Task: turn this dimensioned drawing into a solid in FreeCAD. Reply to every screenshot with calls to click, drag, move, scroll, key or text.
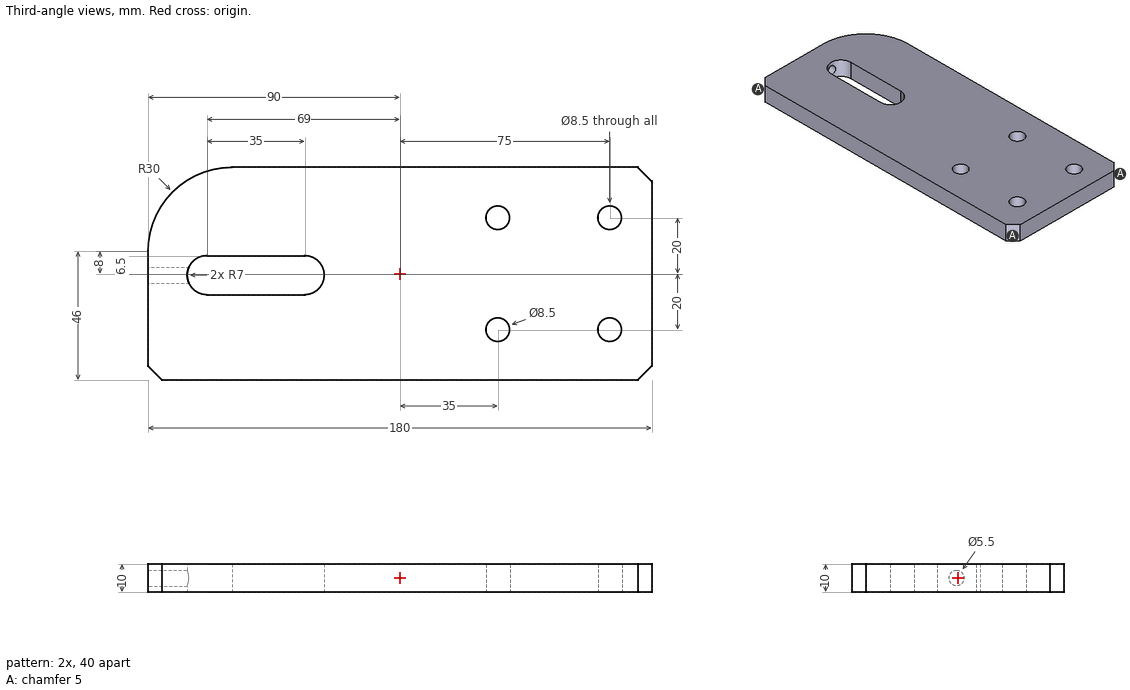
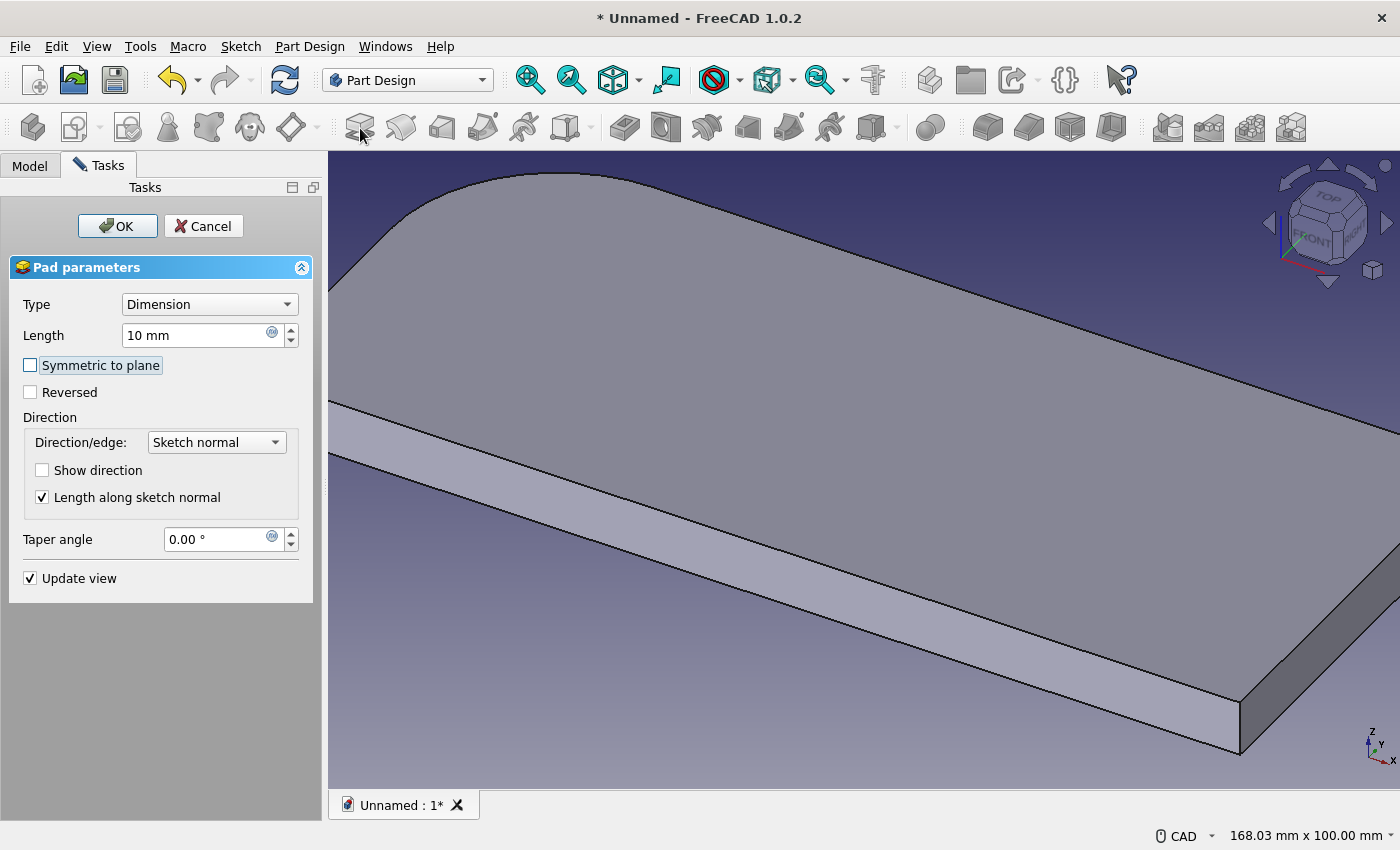
click(31, 365)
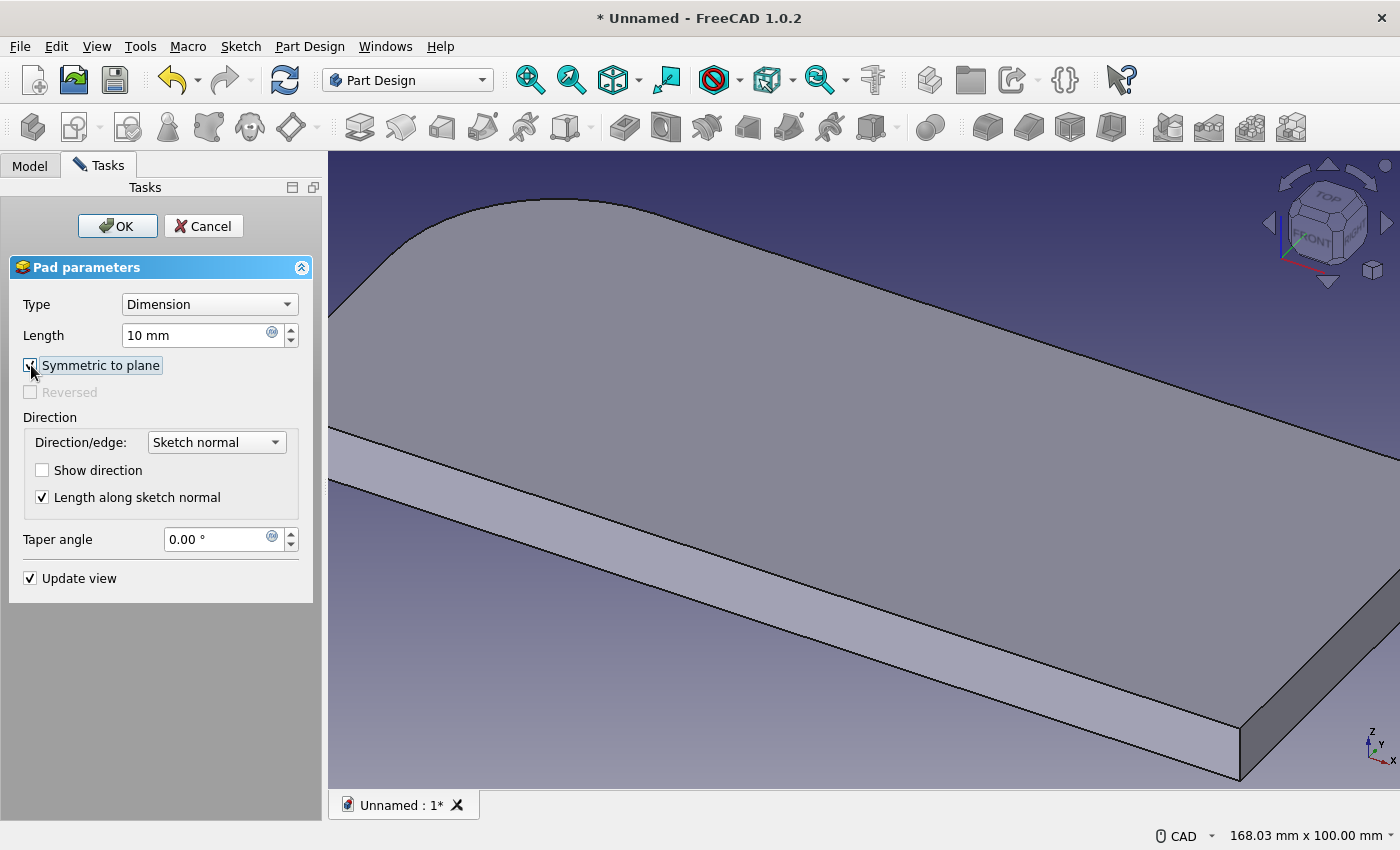
click(118, 226)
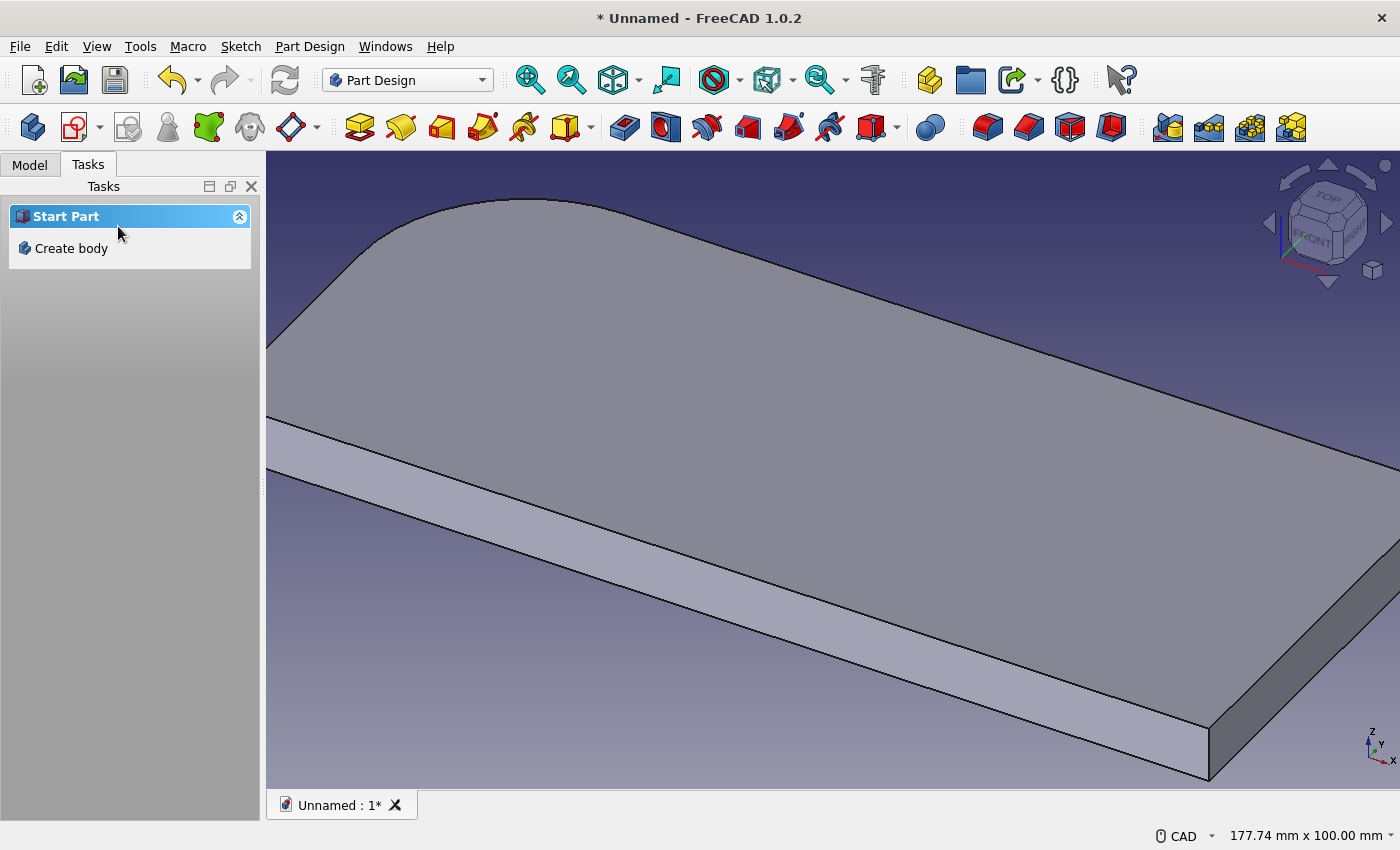
click(531, 80)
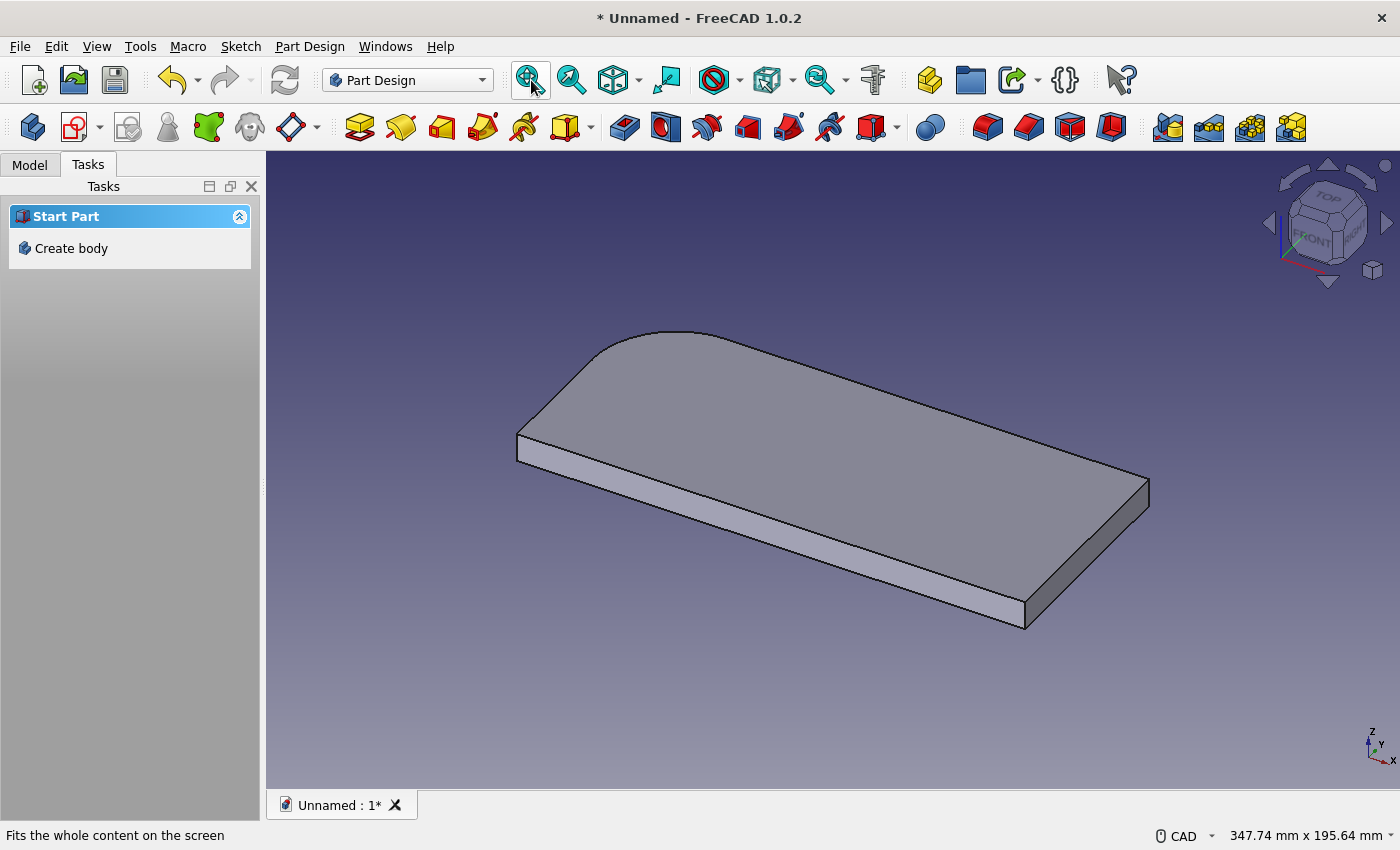
click(978, 504)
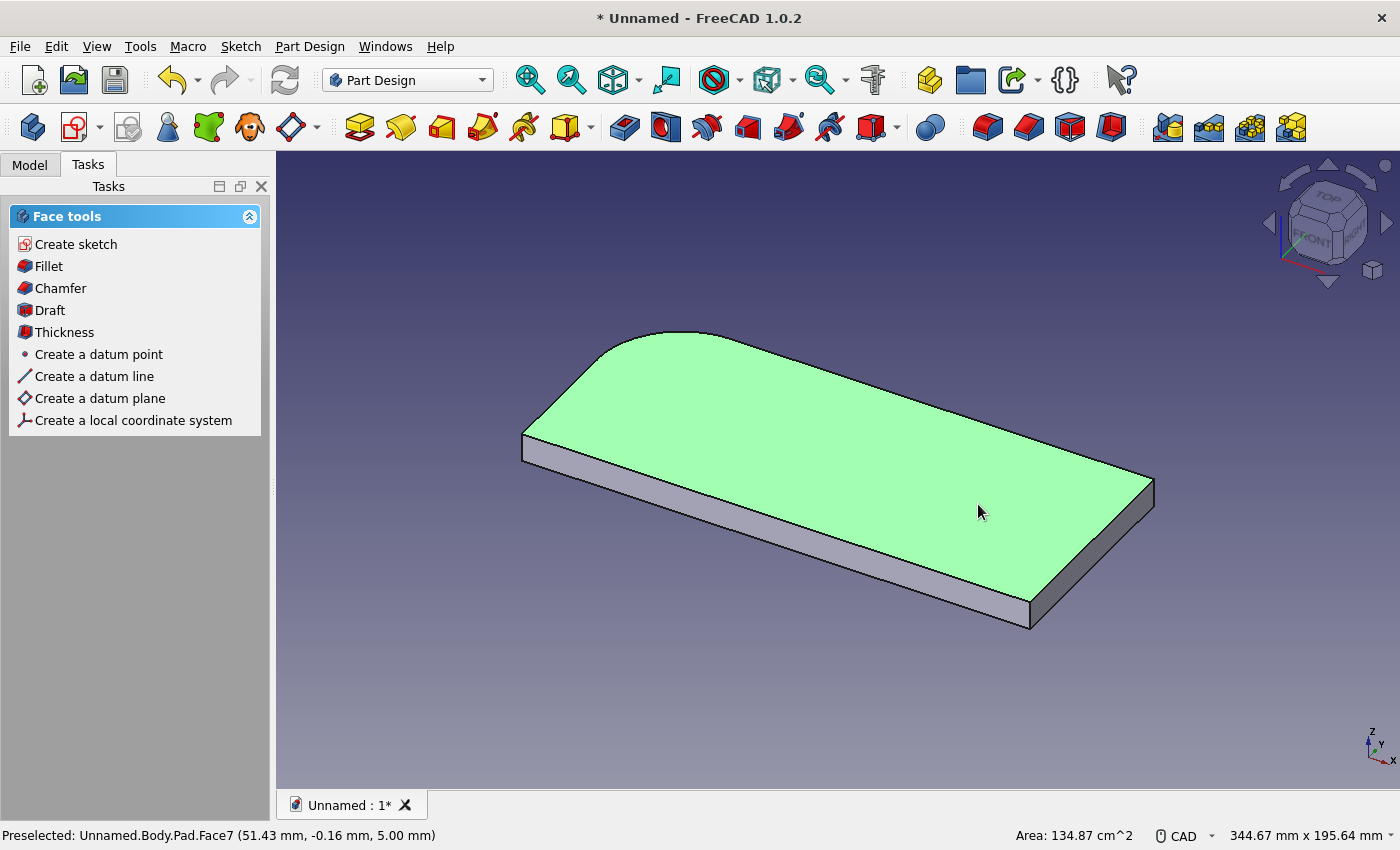
click(74, 128)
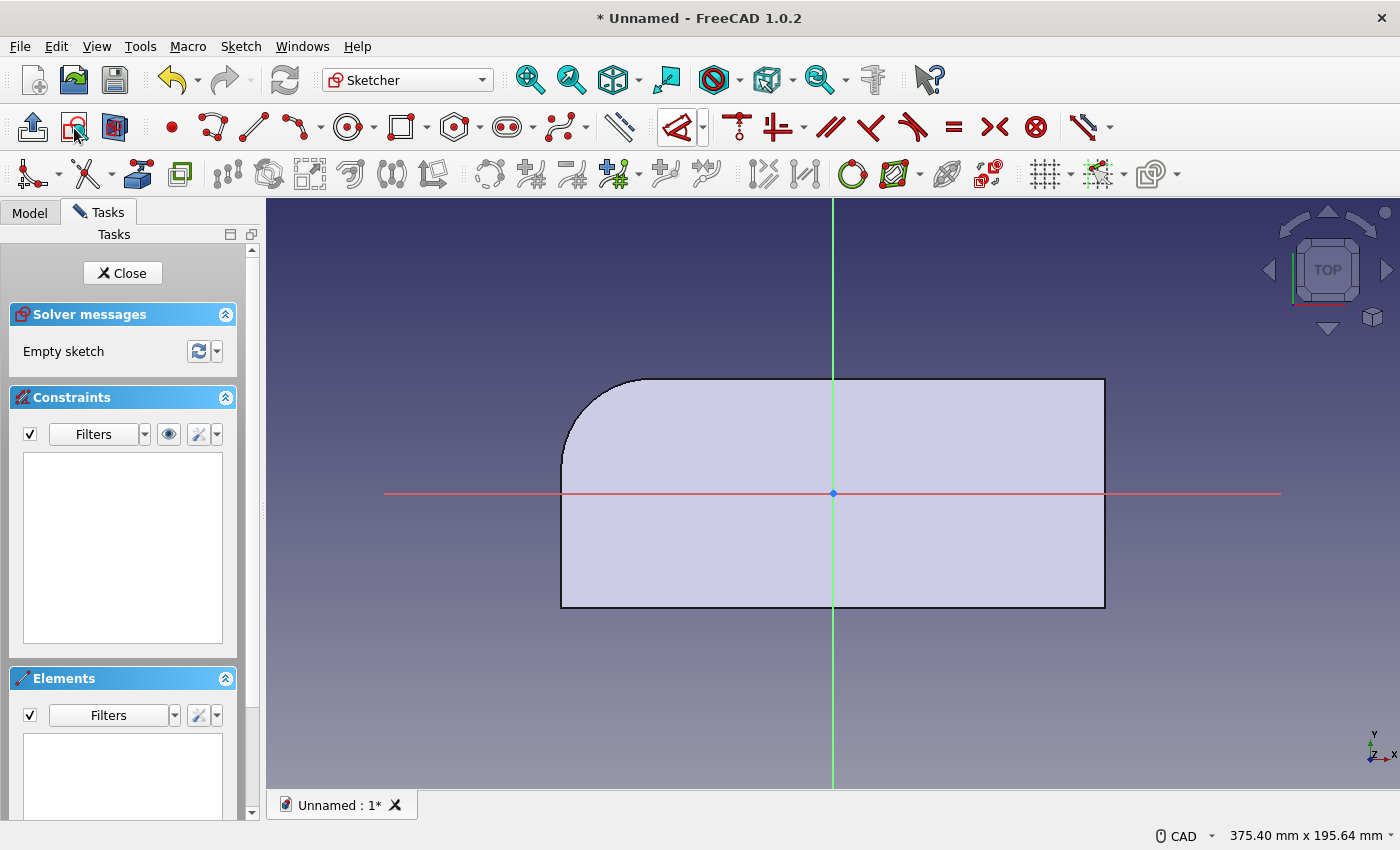
scroll(1083, 428, up, 13)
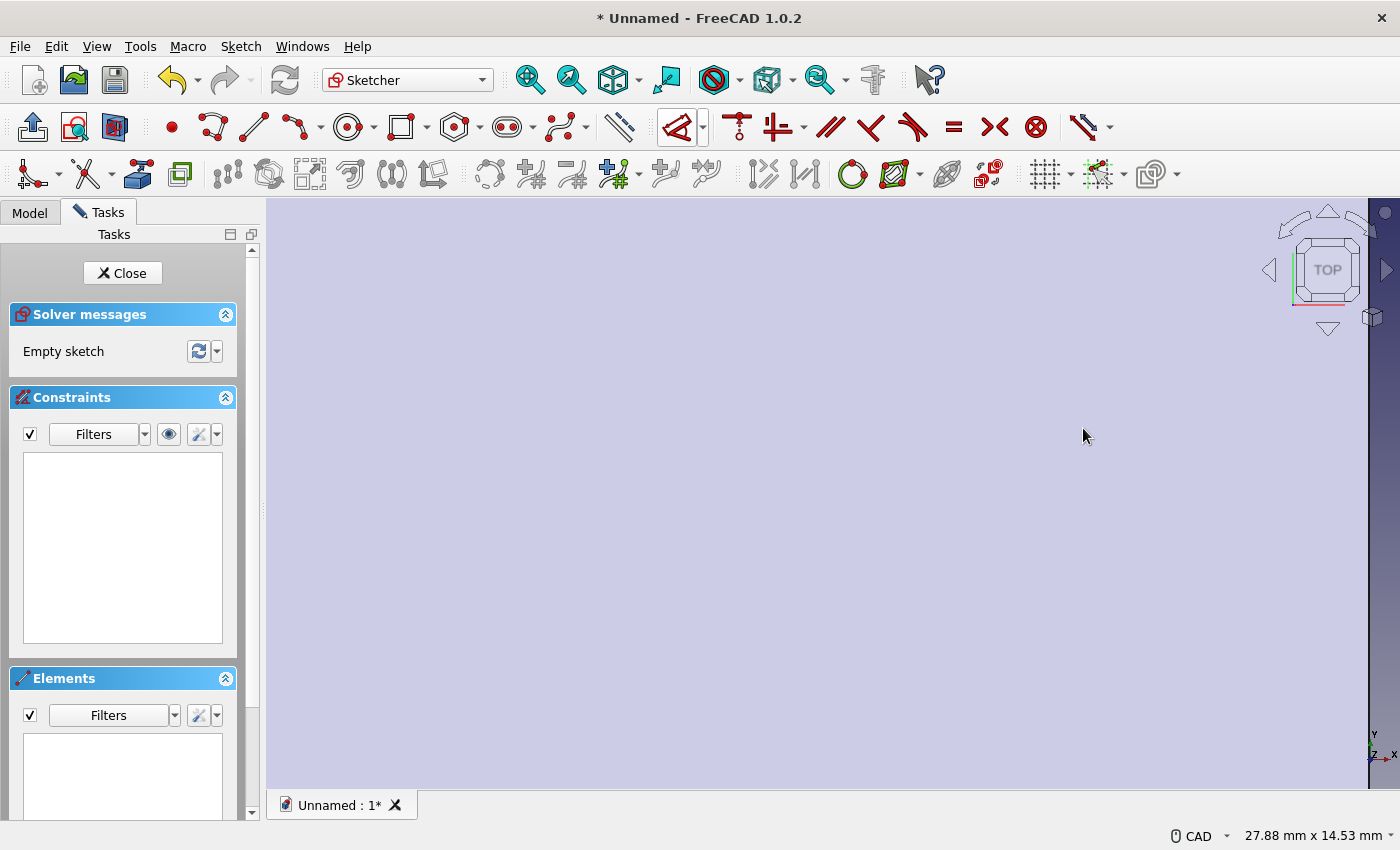
click(348, 128)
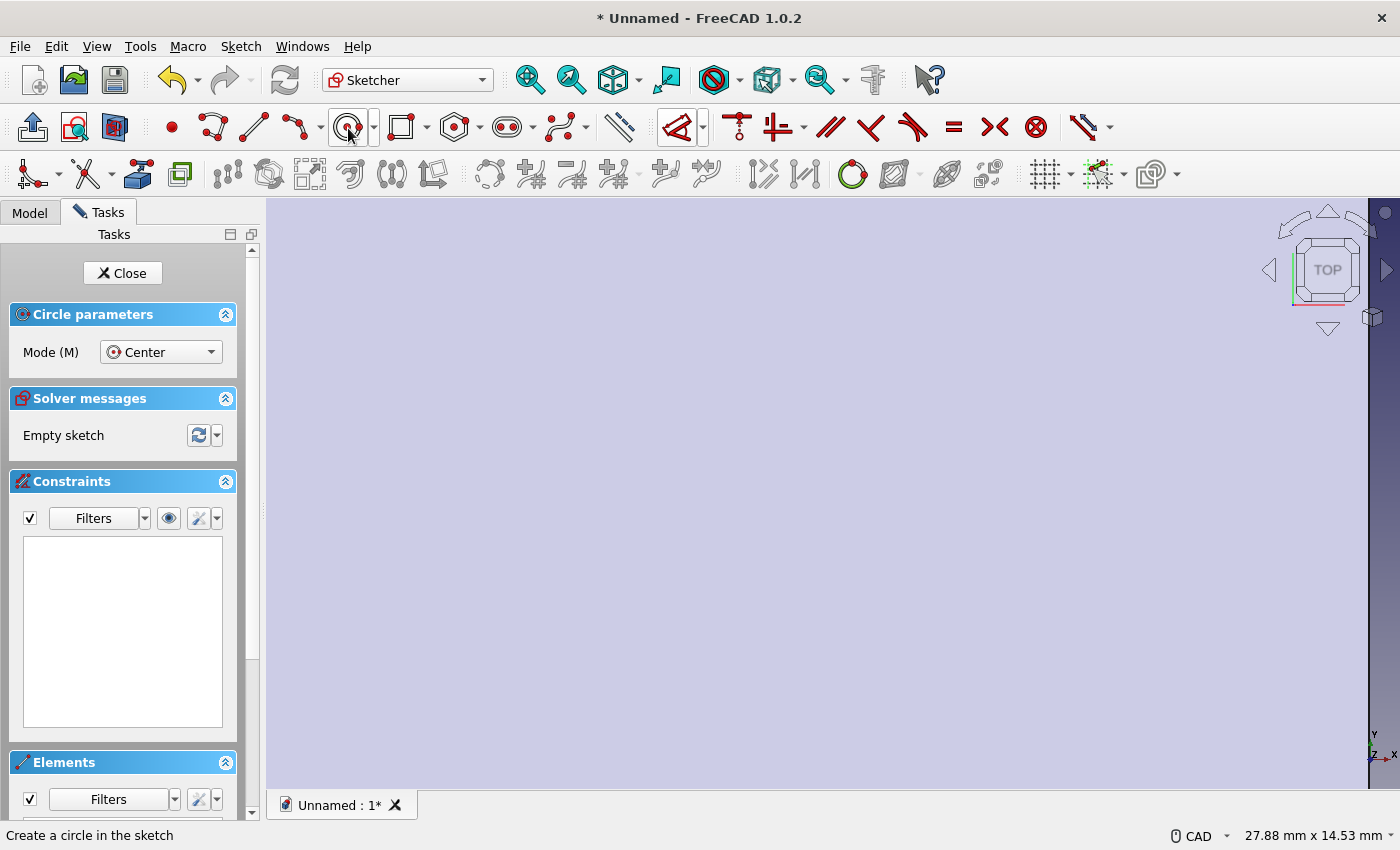
click(758, 492)
click(881, 369)
key(Escape)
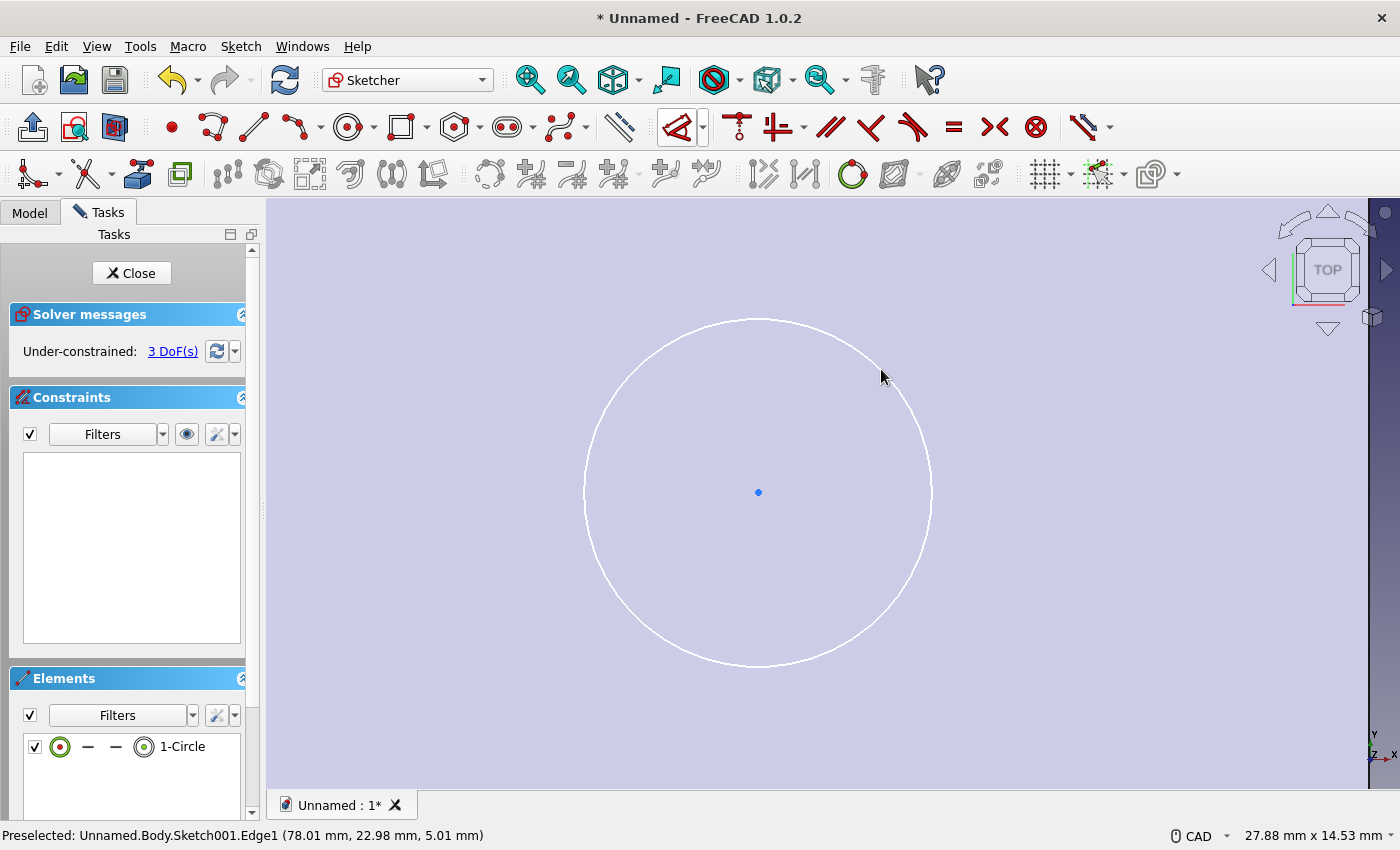
click(881, 370)